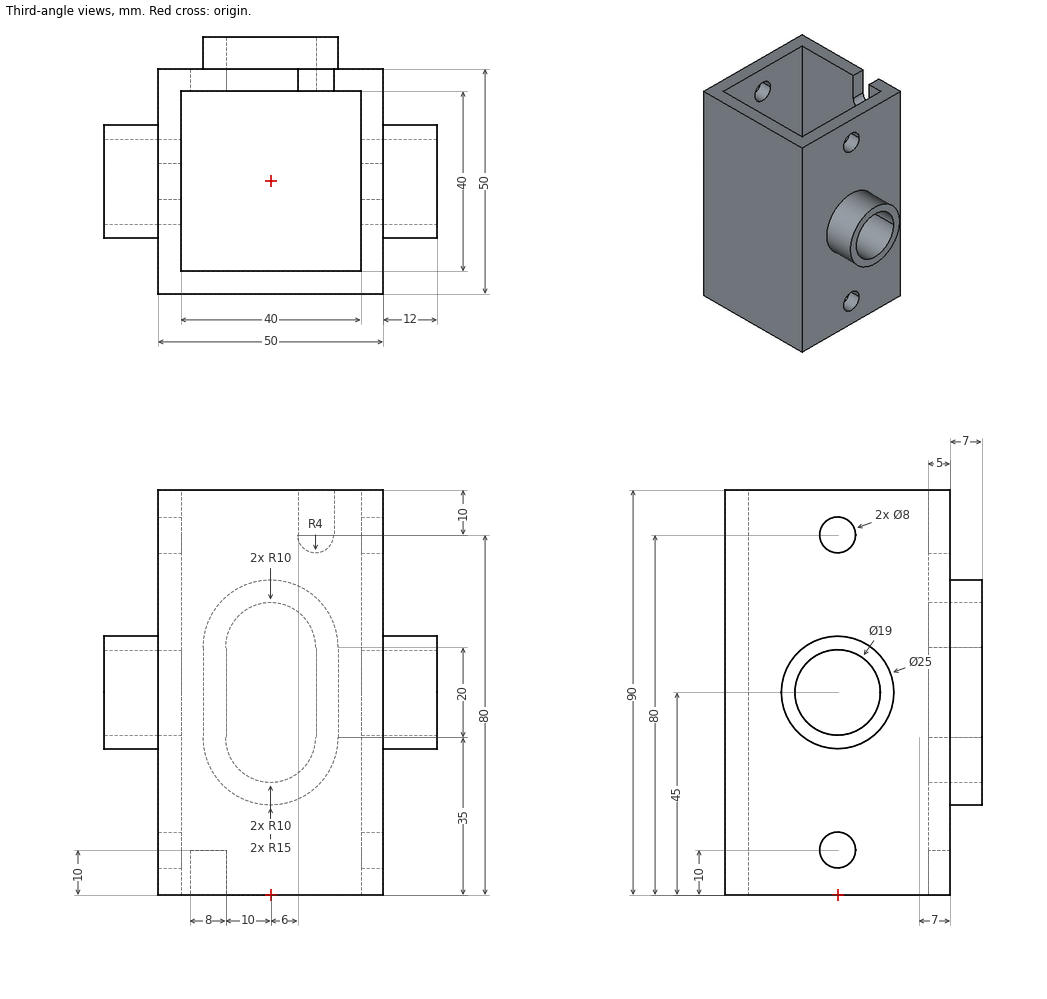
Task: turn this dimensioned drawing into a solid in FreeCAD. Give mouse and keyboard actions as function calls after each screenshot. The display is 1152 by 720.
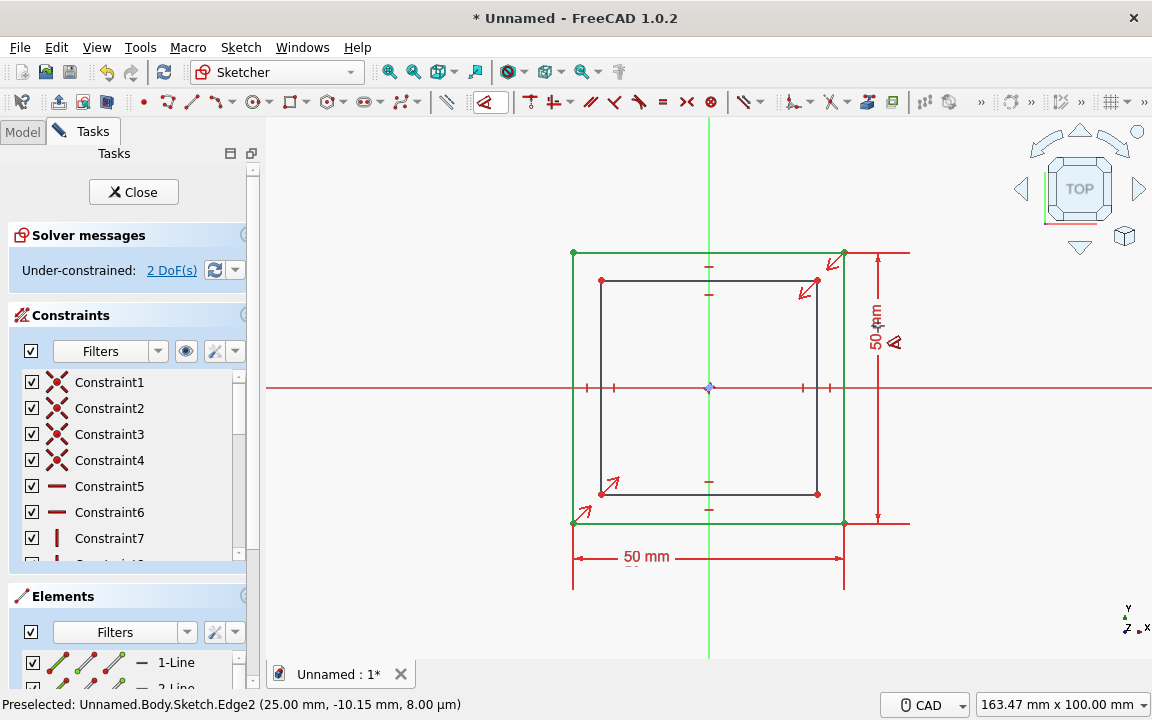
click(666, 495)
click(659, 461)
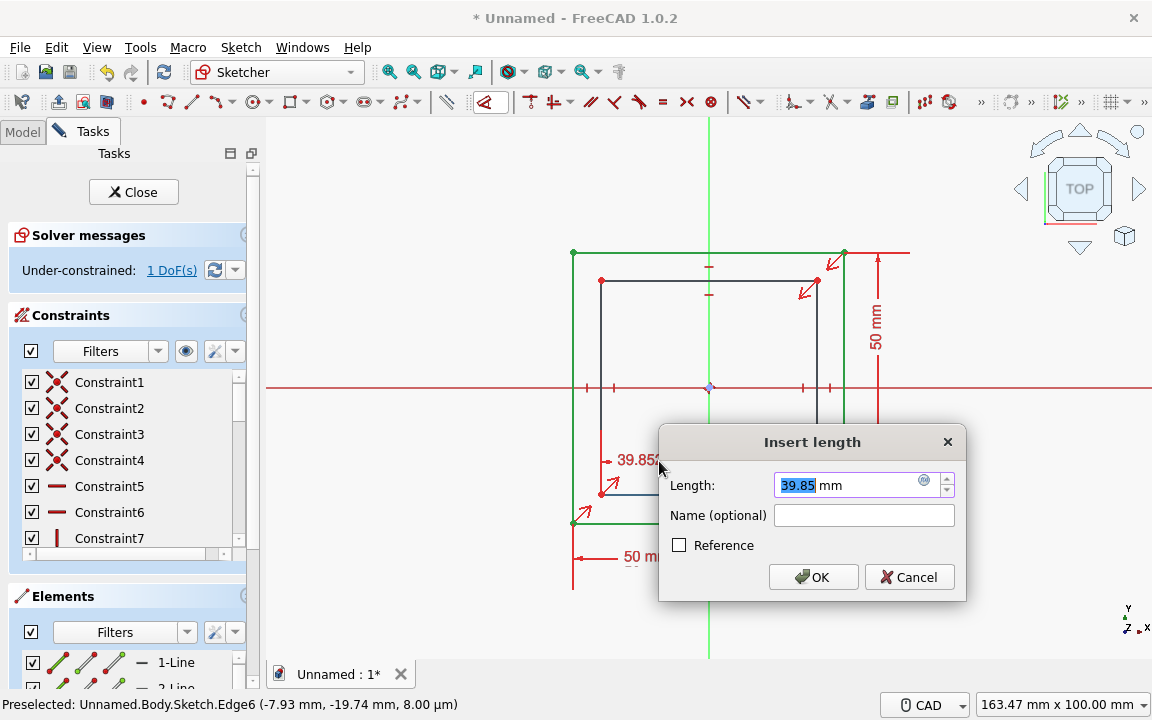
text(40)
key(Return)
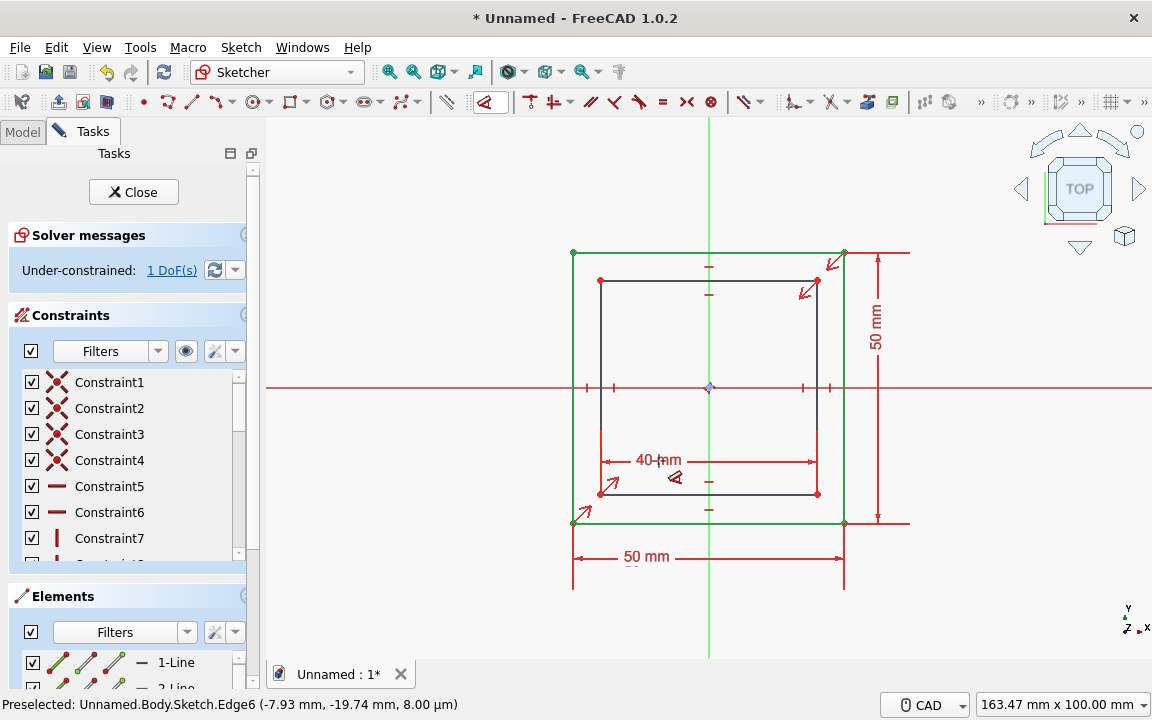
click(817, 431)
click(783, 339)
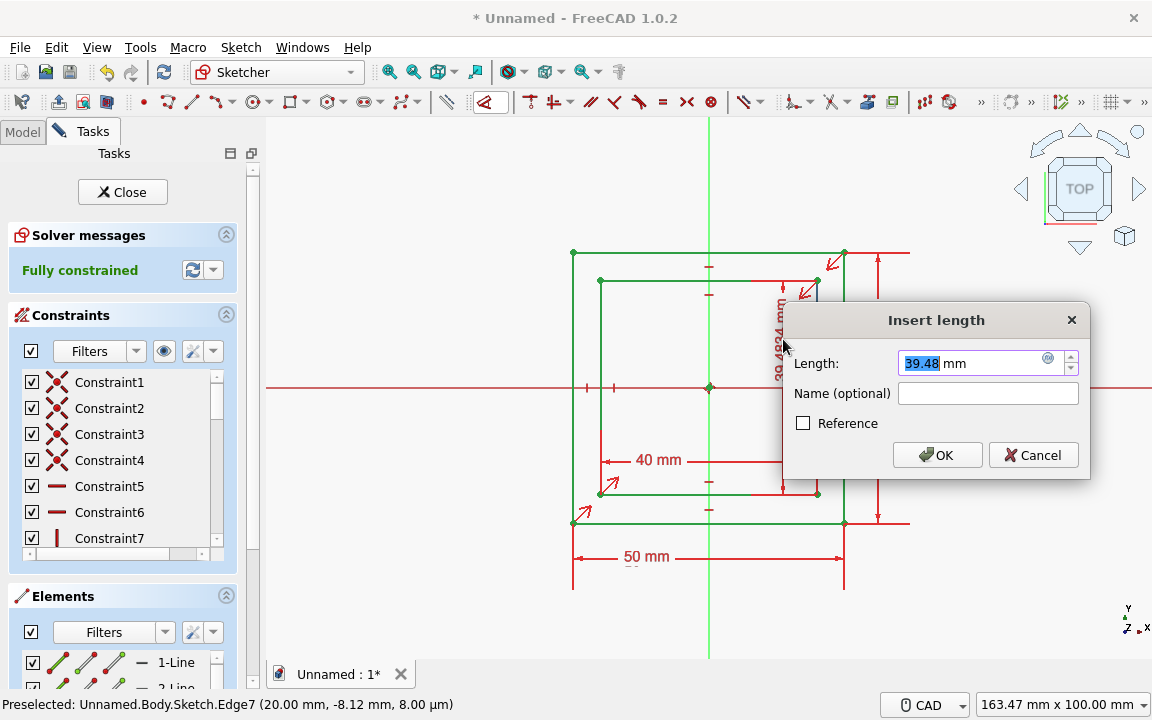
text(40)
key(Return)
key(Escape)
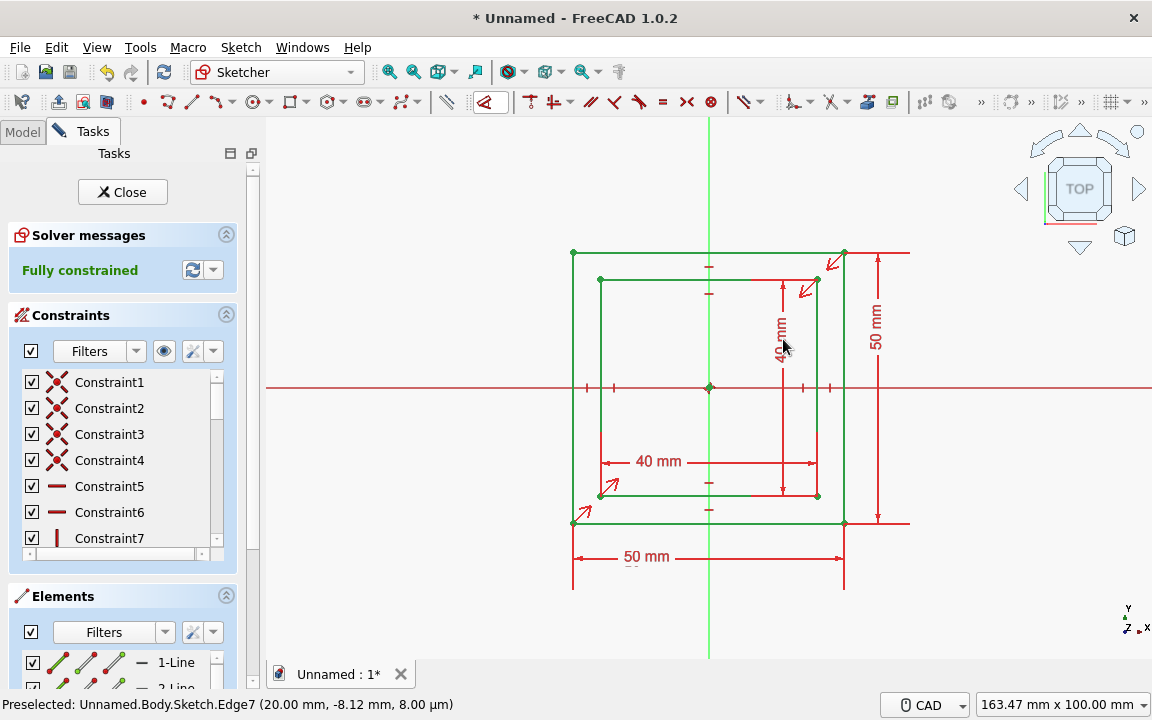
click(123, 192)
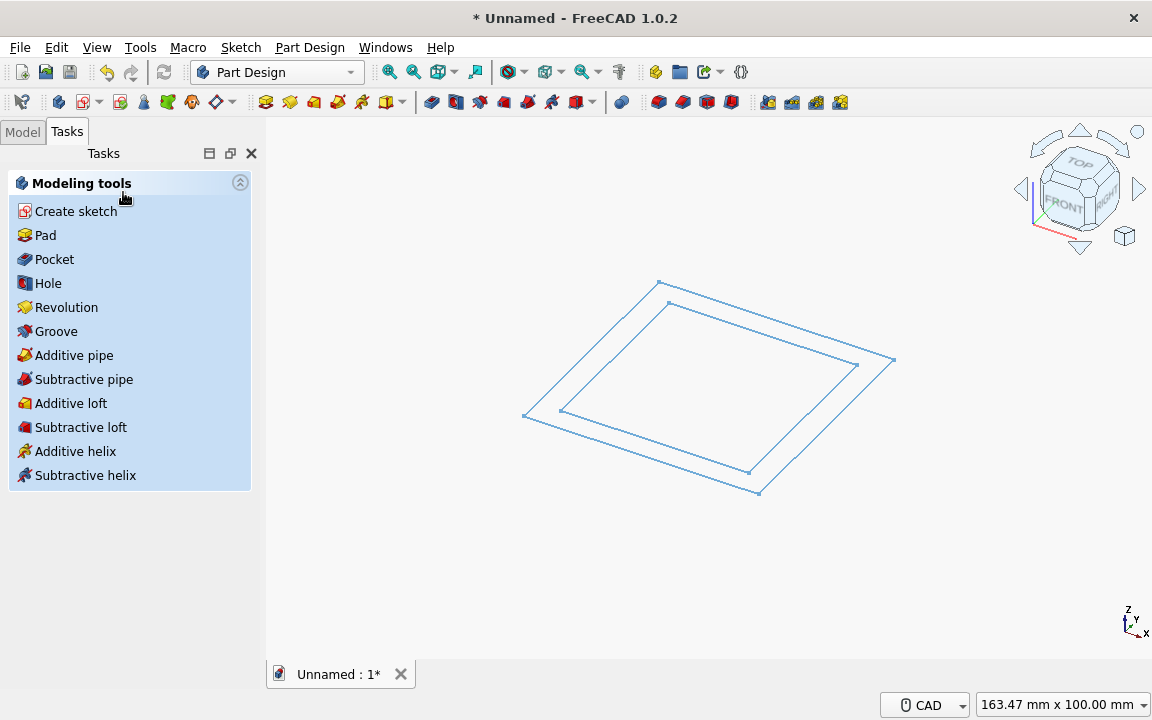
click(266, 102)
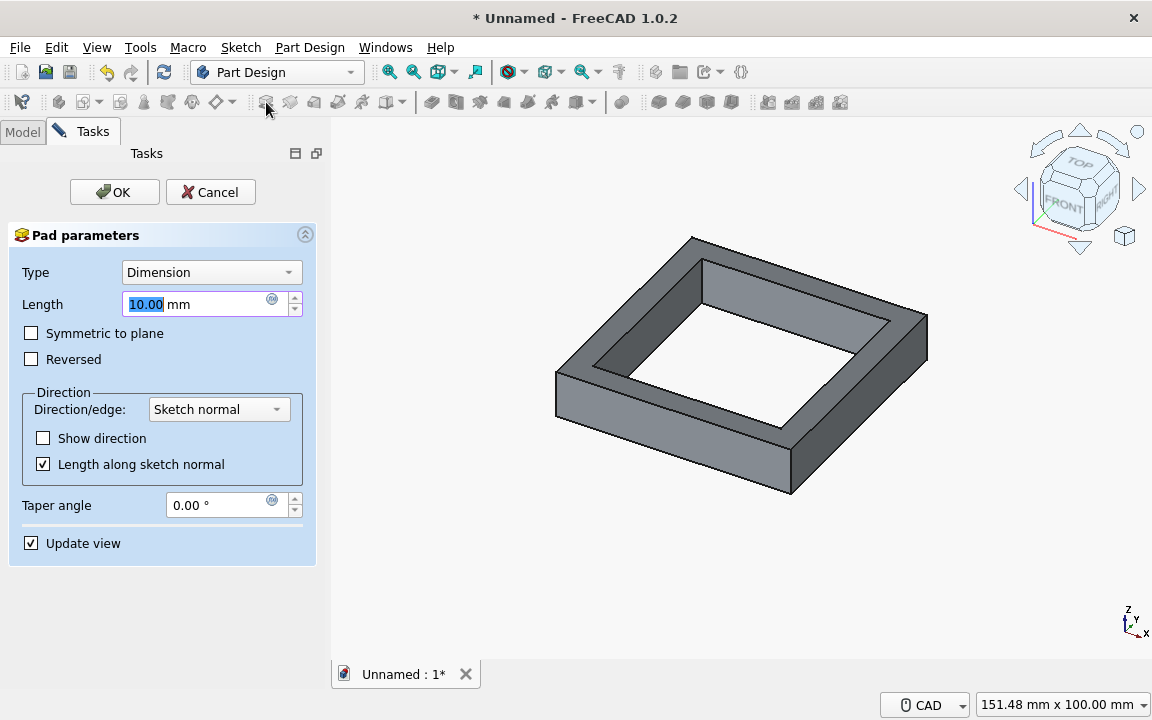
text(90)
key(Tab)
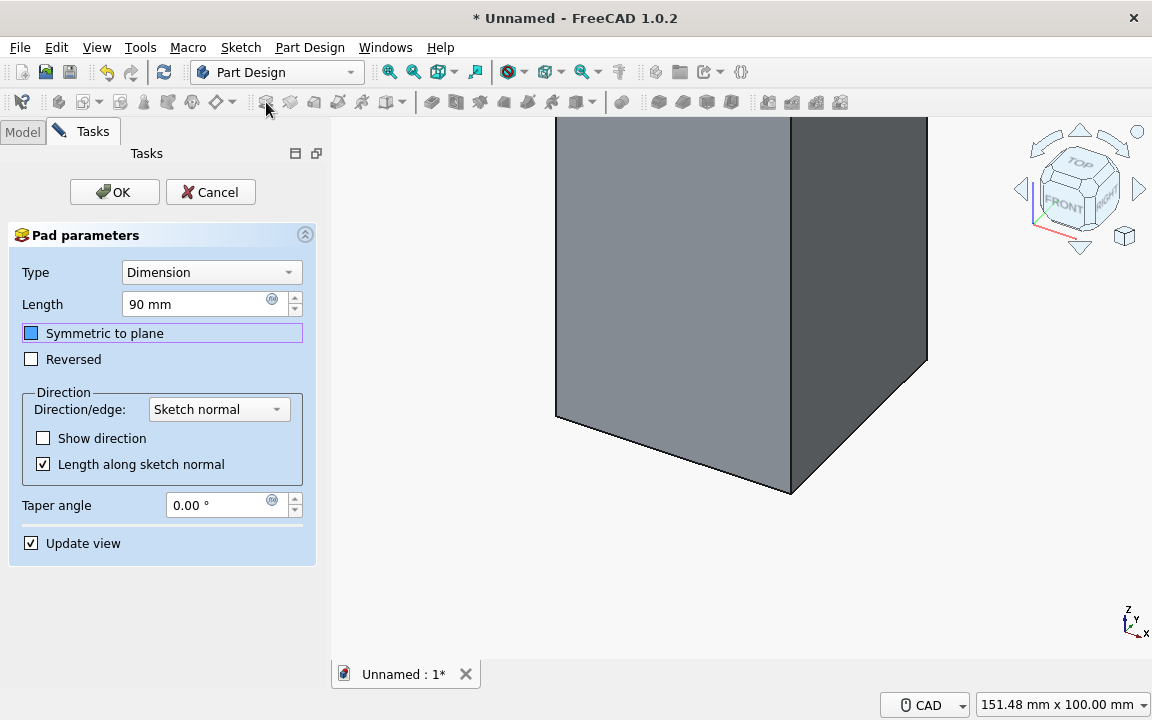
click(115, 192)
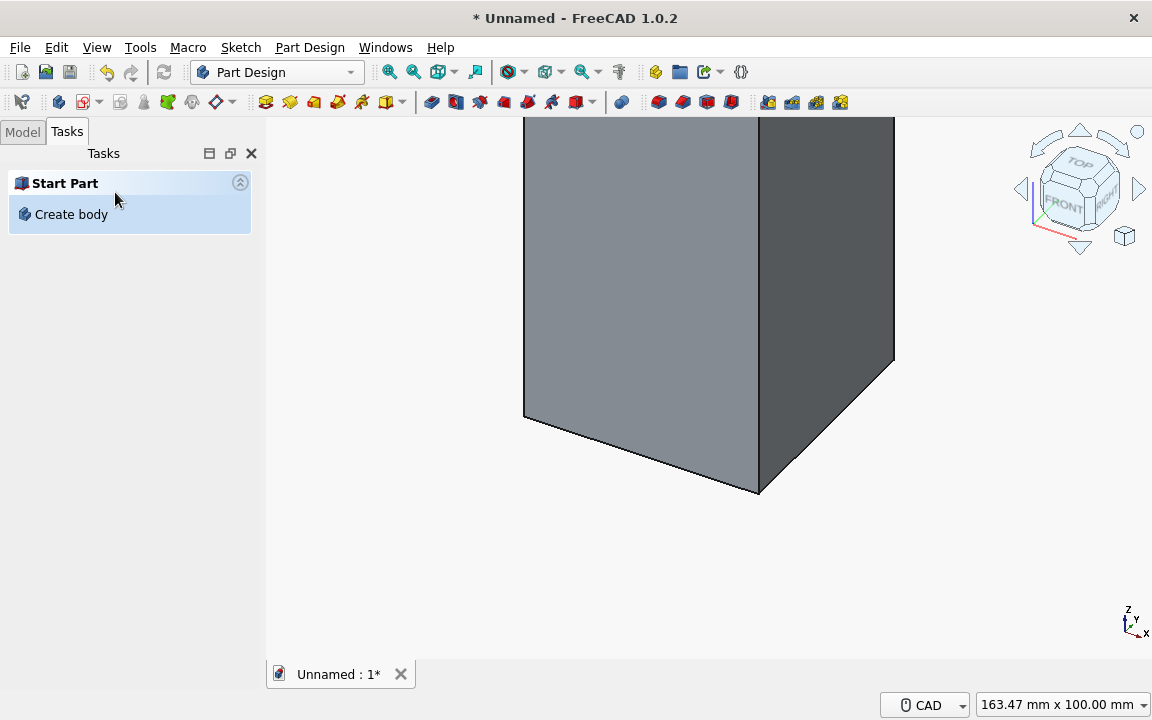
key(v)
key(f)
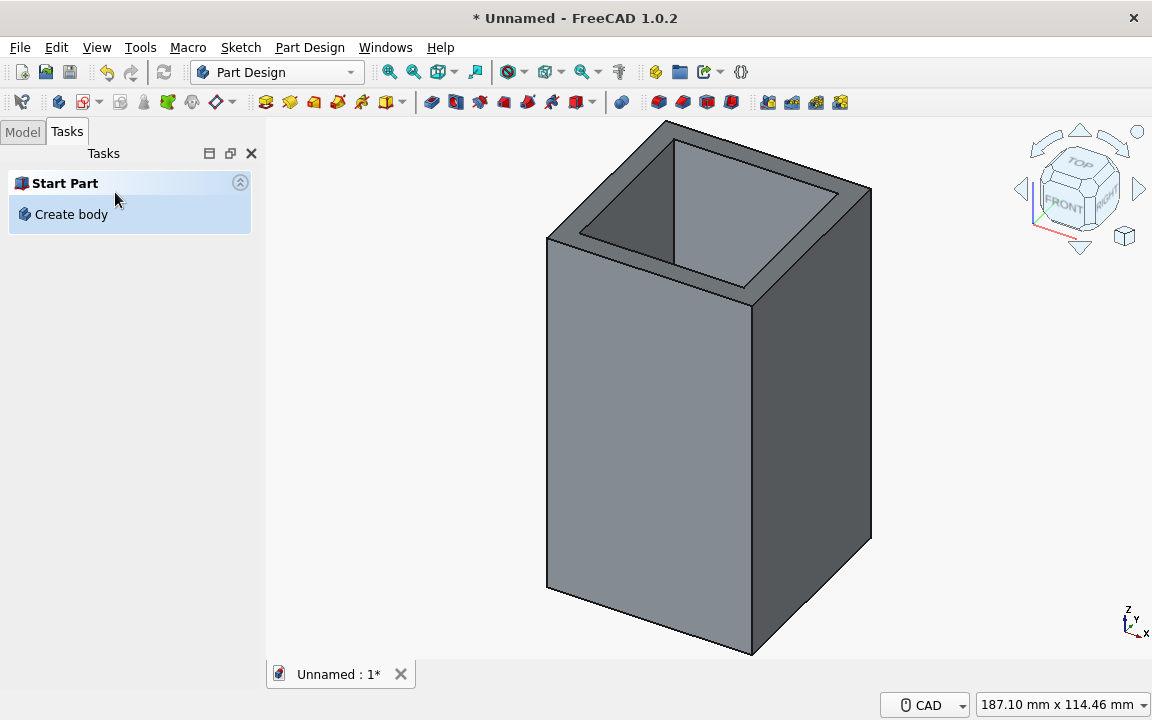
key(4)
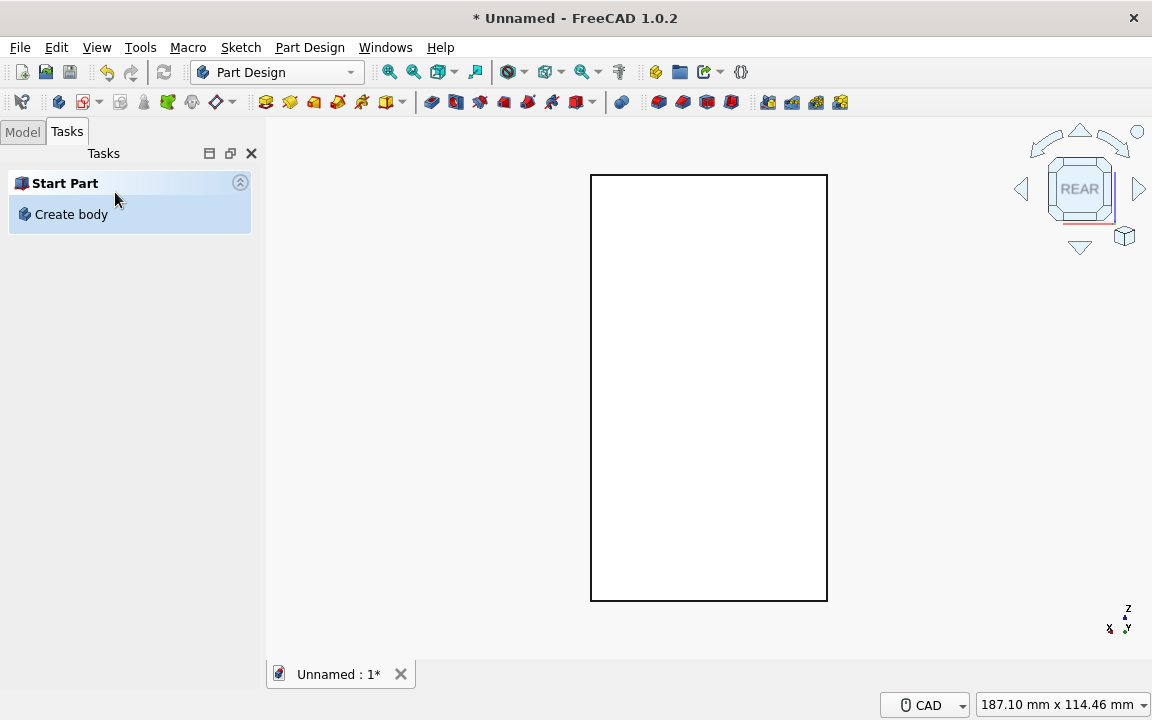
click(709, 326)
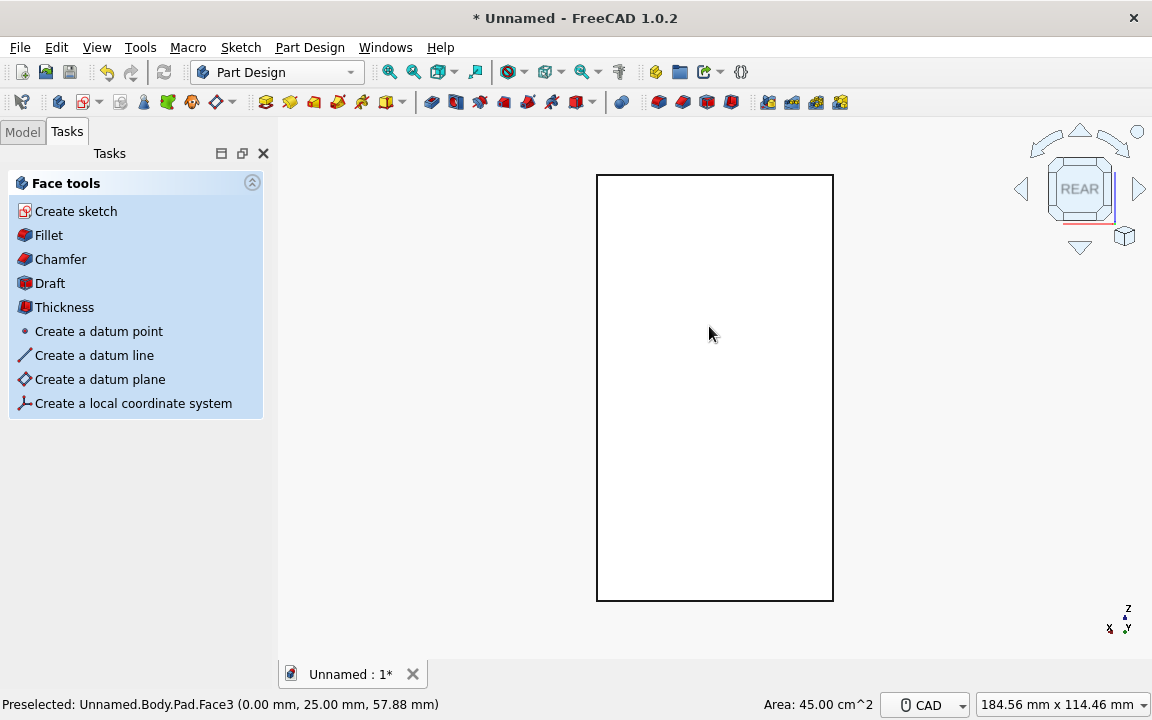
click(84, 102)